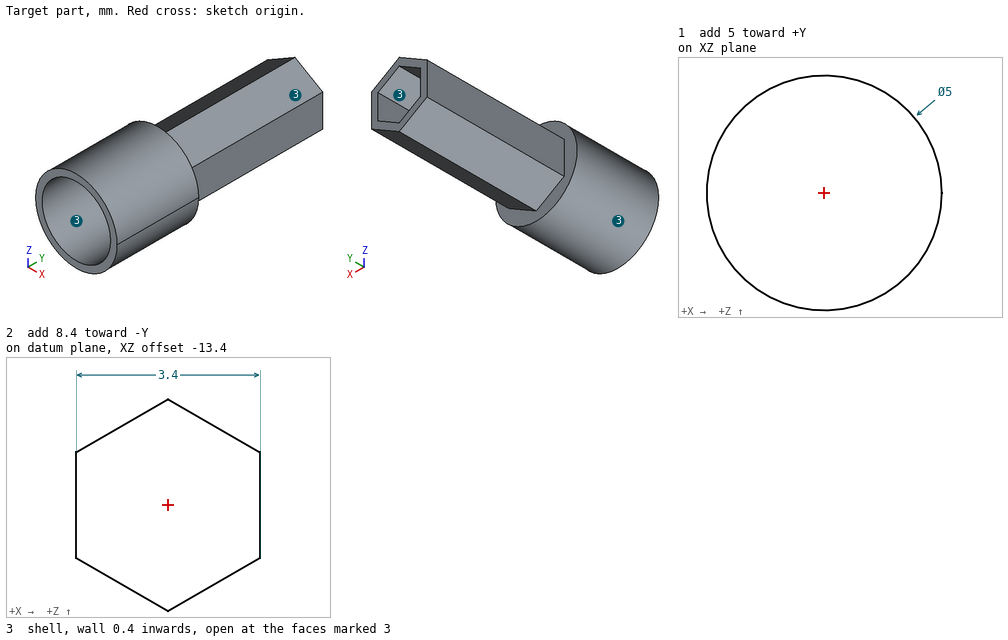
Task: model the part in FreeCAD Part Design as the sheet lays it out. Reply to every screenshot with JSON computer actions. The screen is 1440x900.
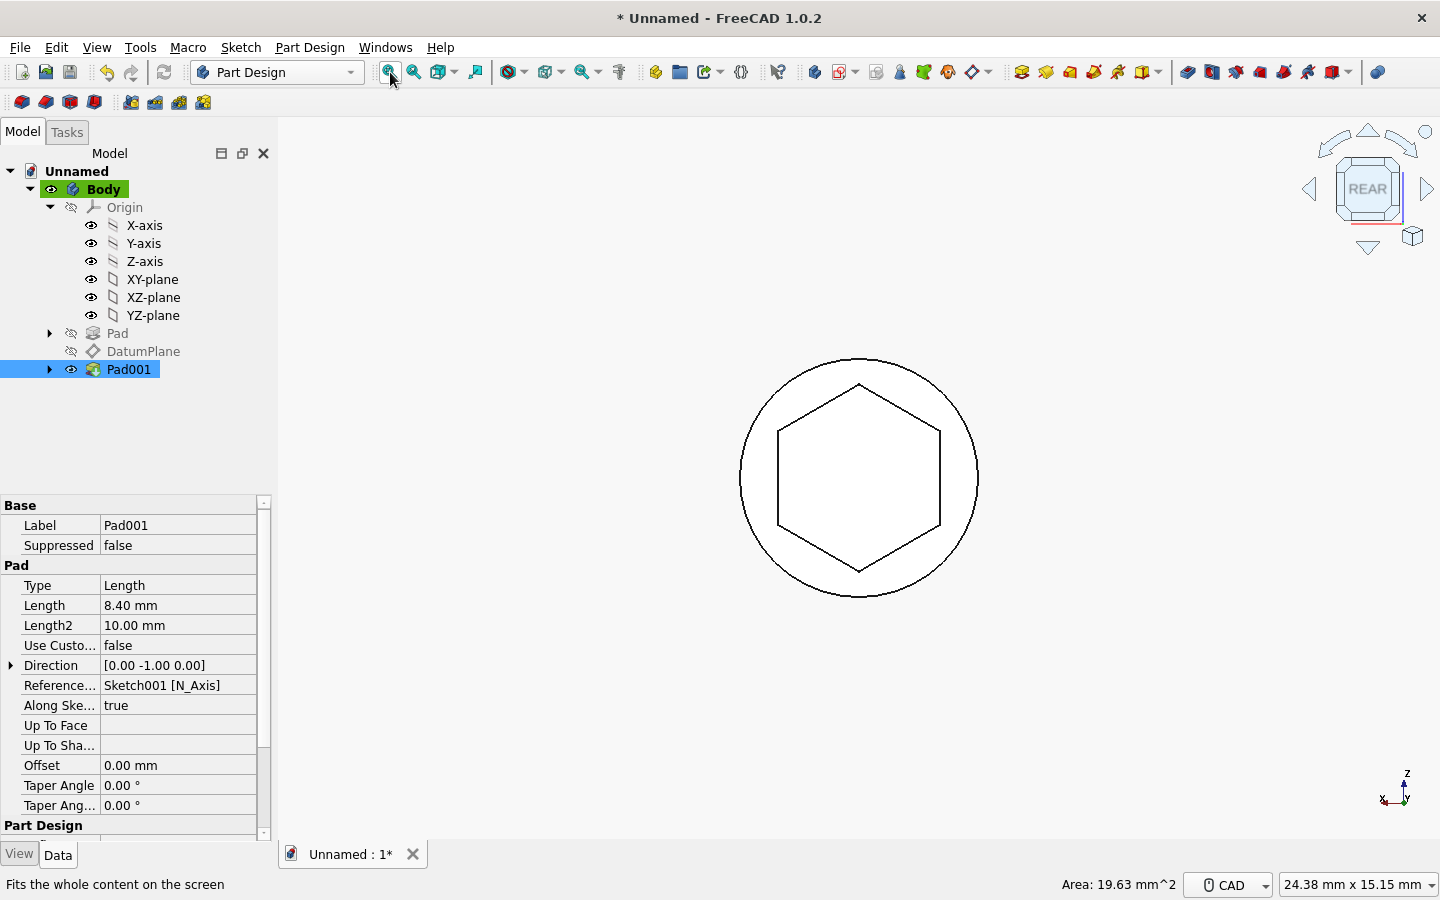
{"action": "left_click", "coordinate": [859, 477], "text": "ctrl"}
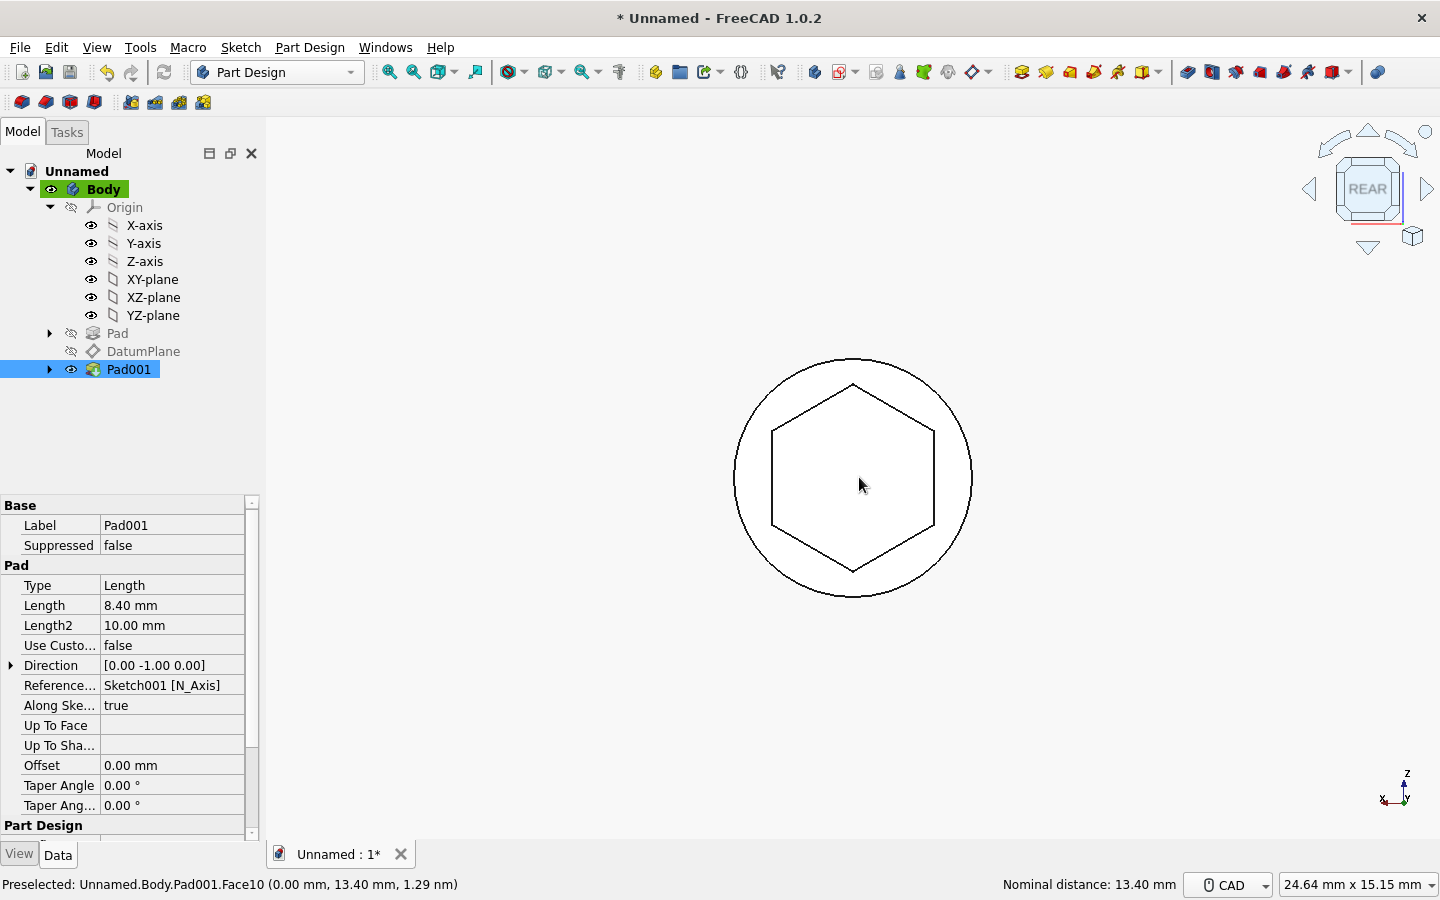
{"action": "left_click", "coordinate": [94, 102]}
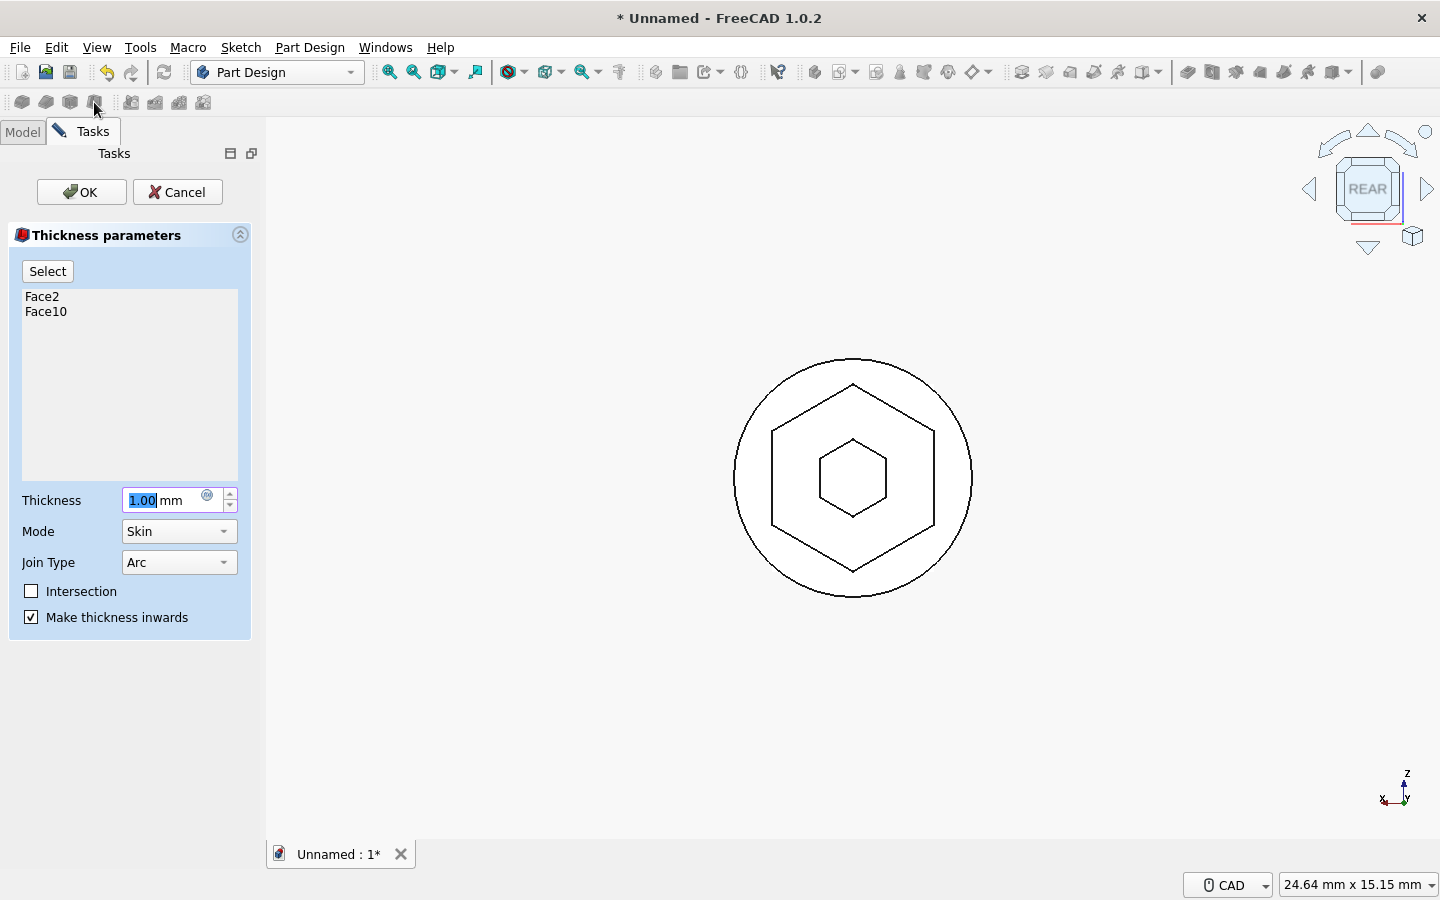
{"action": "type", "text": "0.4"}
{"action": "key", "text": "Tab"}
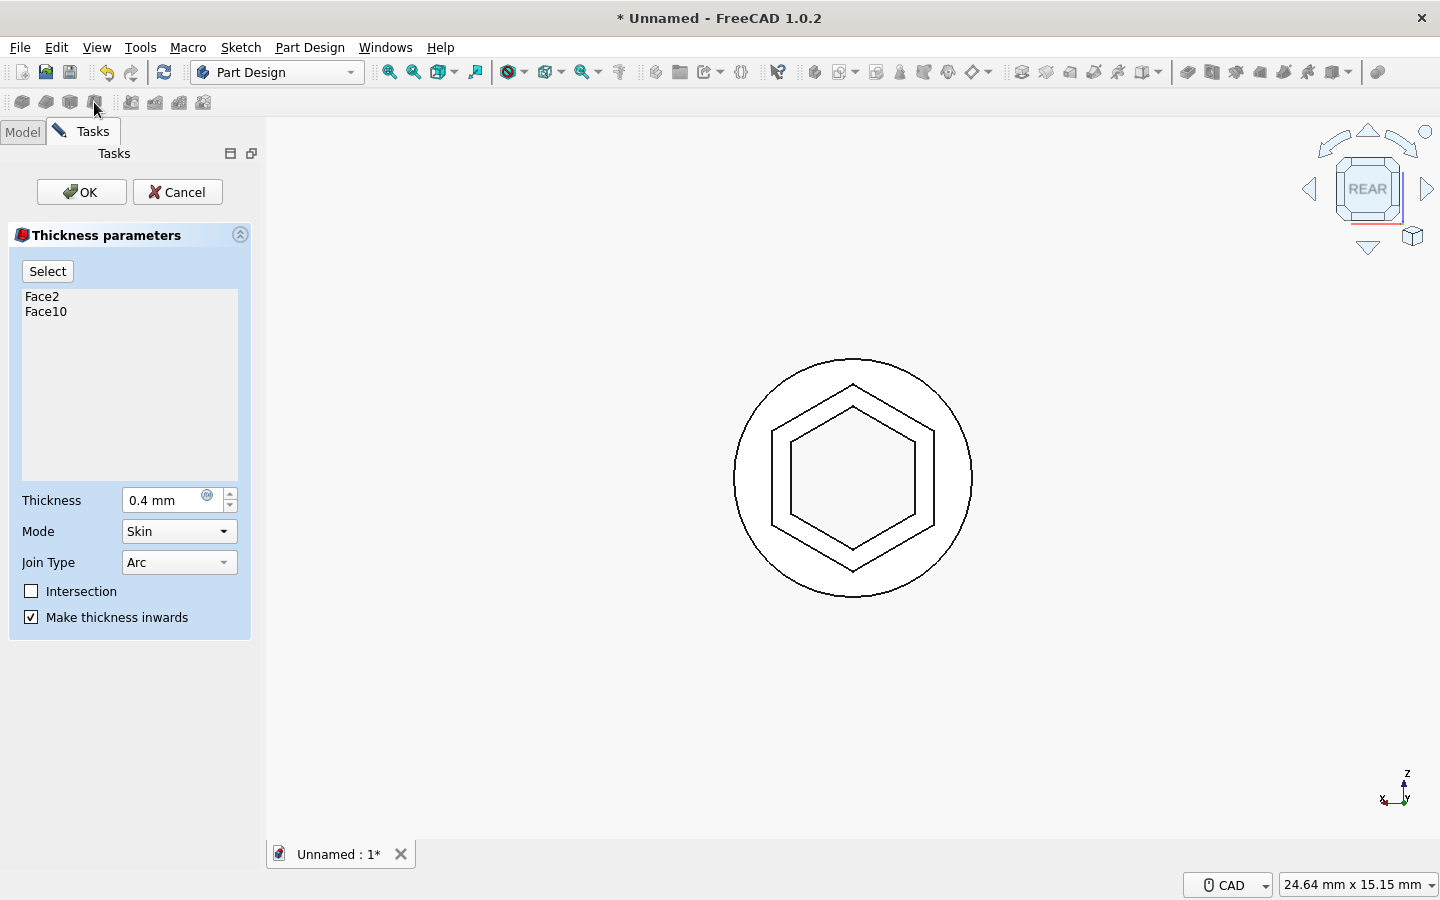
{"action": "left_click", "coordinate": [180, 562]}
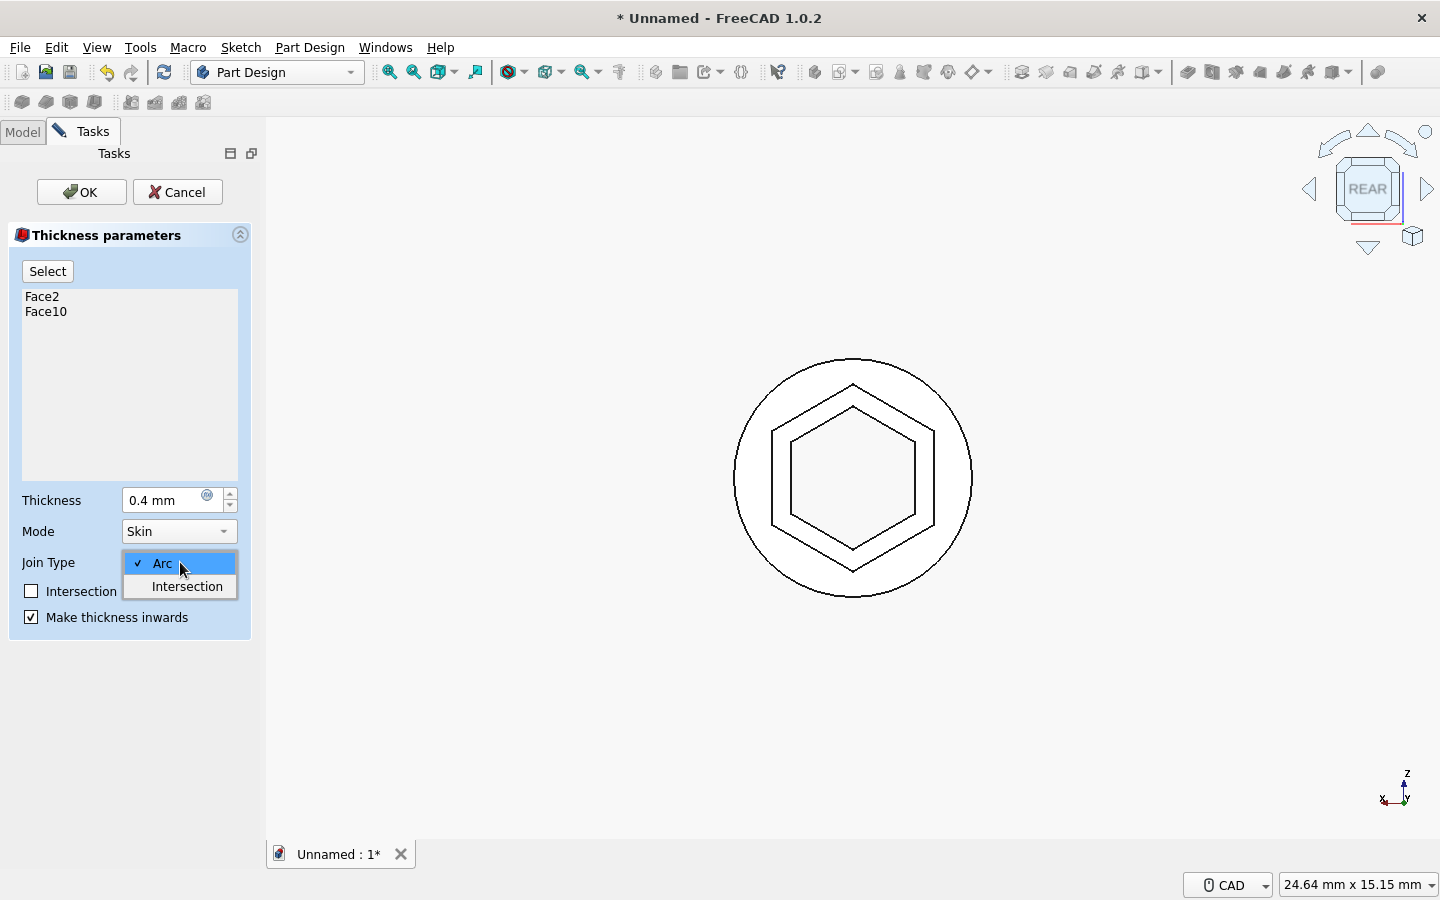
{"action": "left_click", "coordinate": [179, 586]}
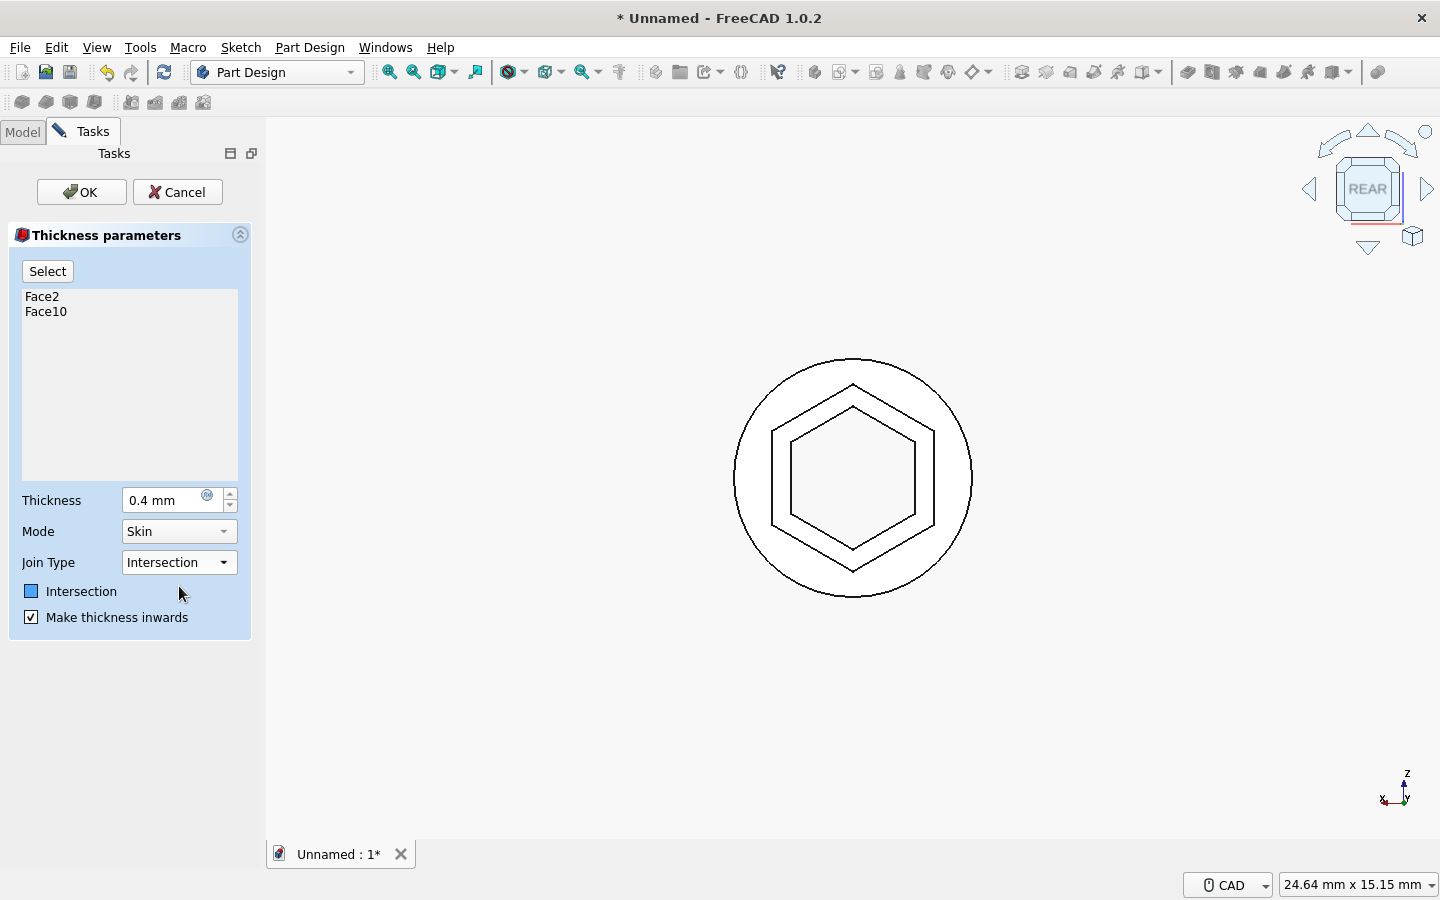
{"action": "left_click", "coordinate": [82, 192]}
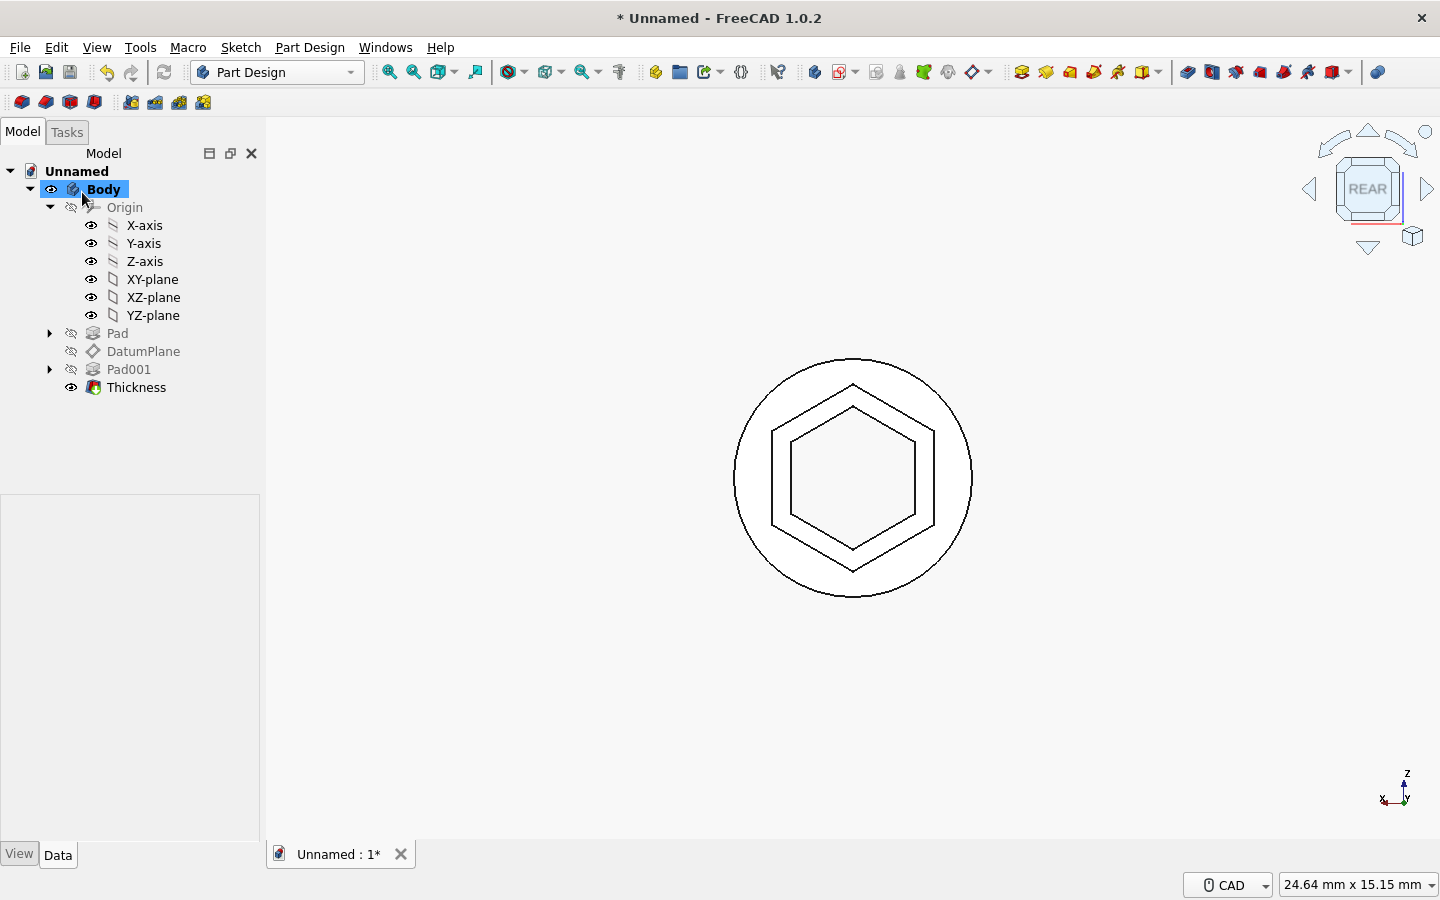
{"action": "key", "text": "0"}